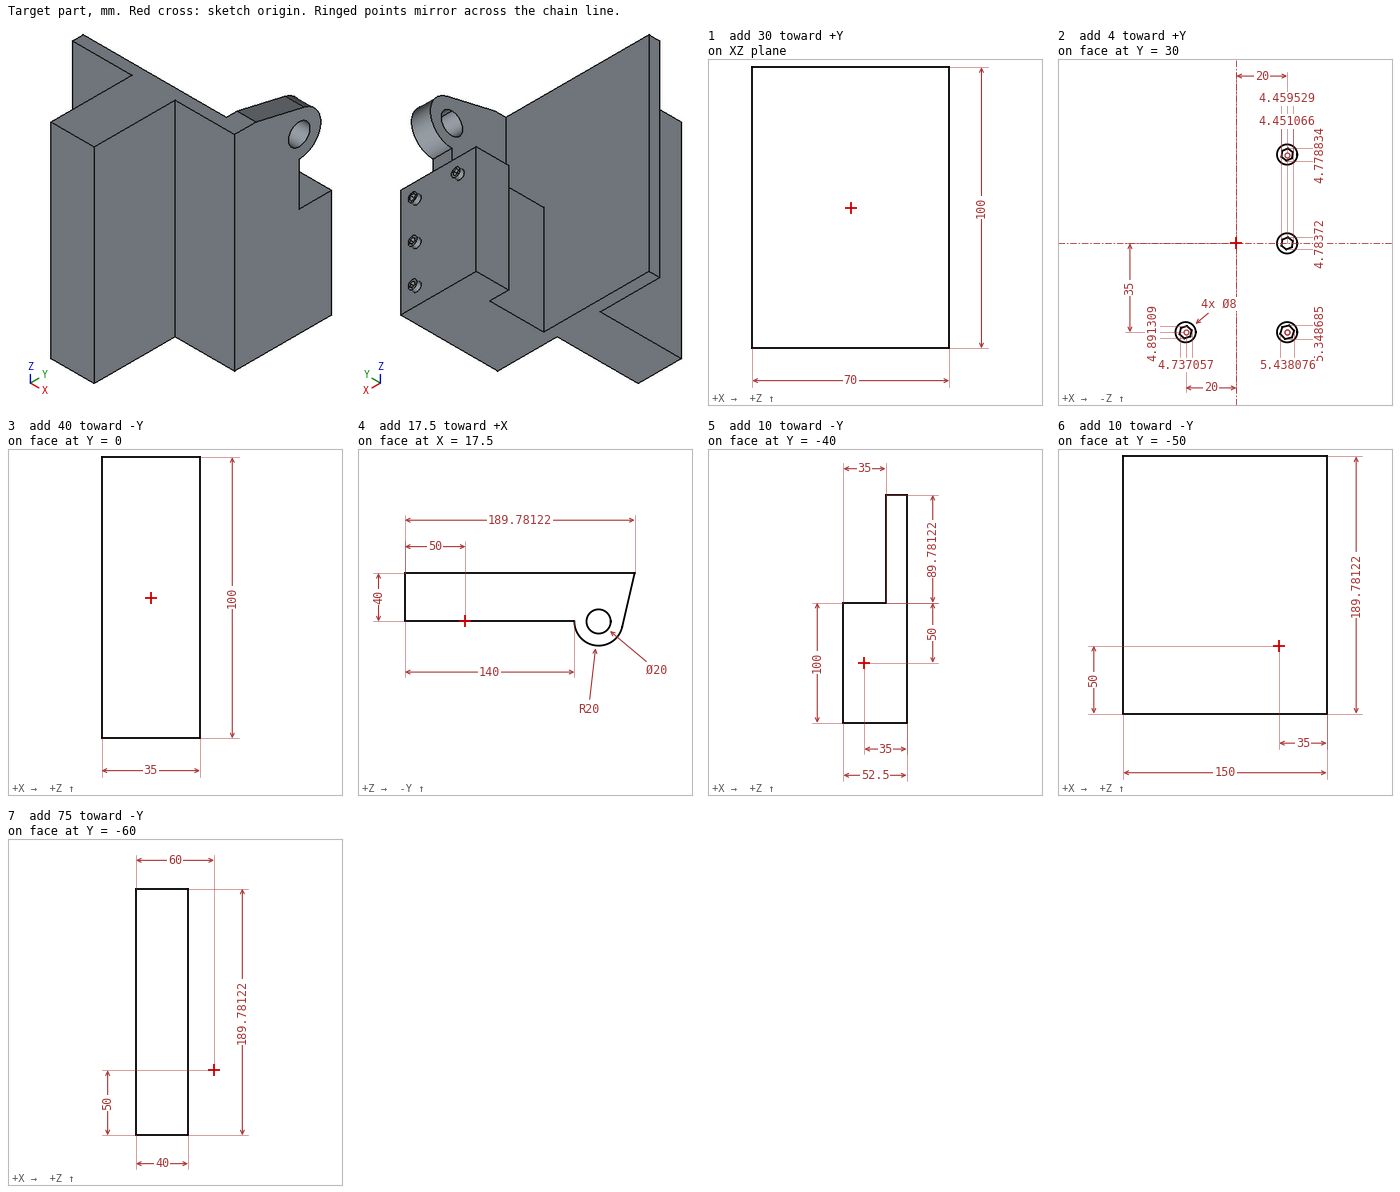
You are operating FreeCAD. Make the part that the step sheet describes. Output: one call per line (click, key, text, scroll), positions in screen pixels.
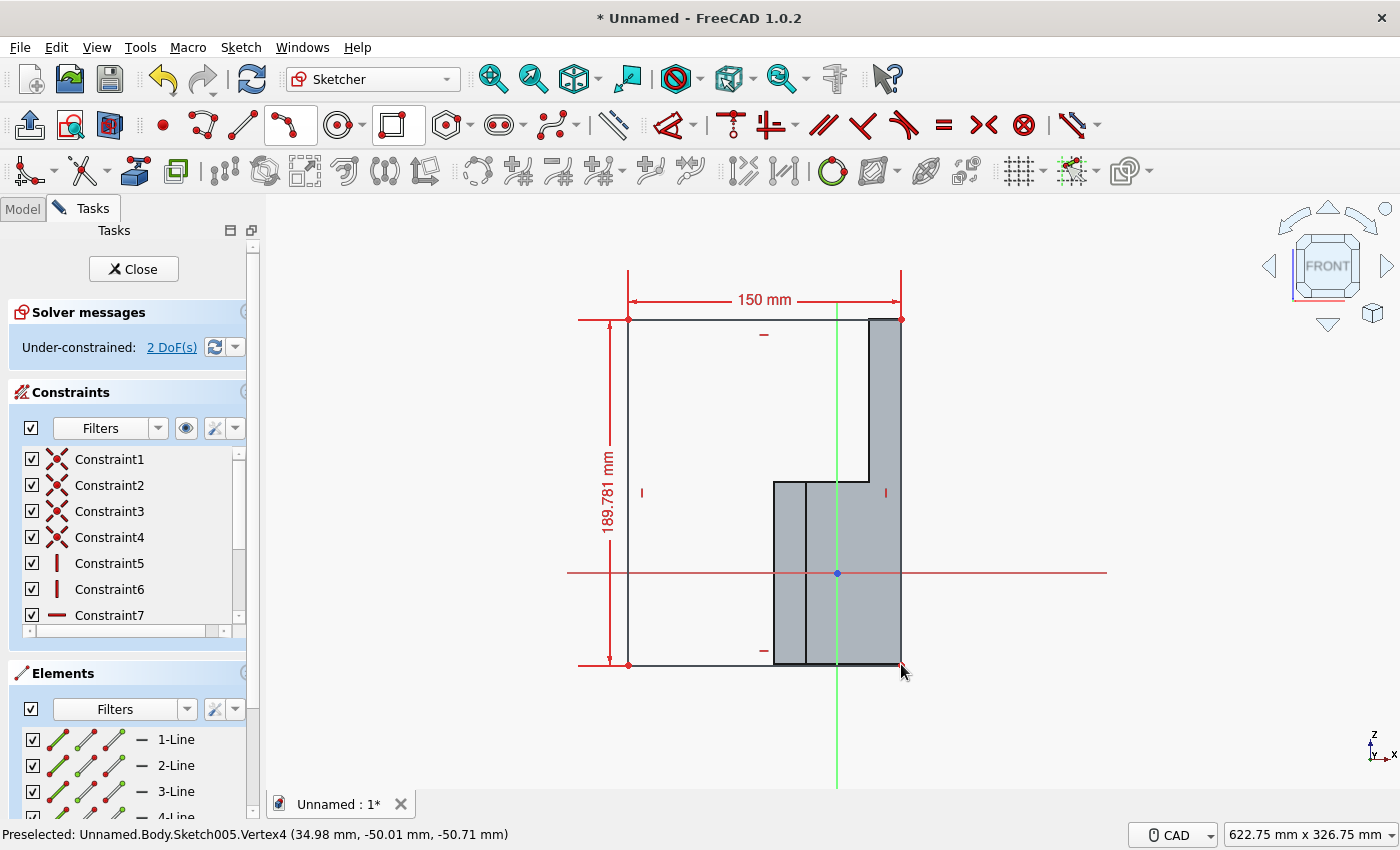
key(d)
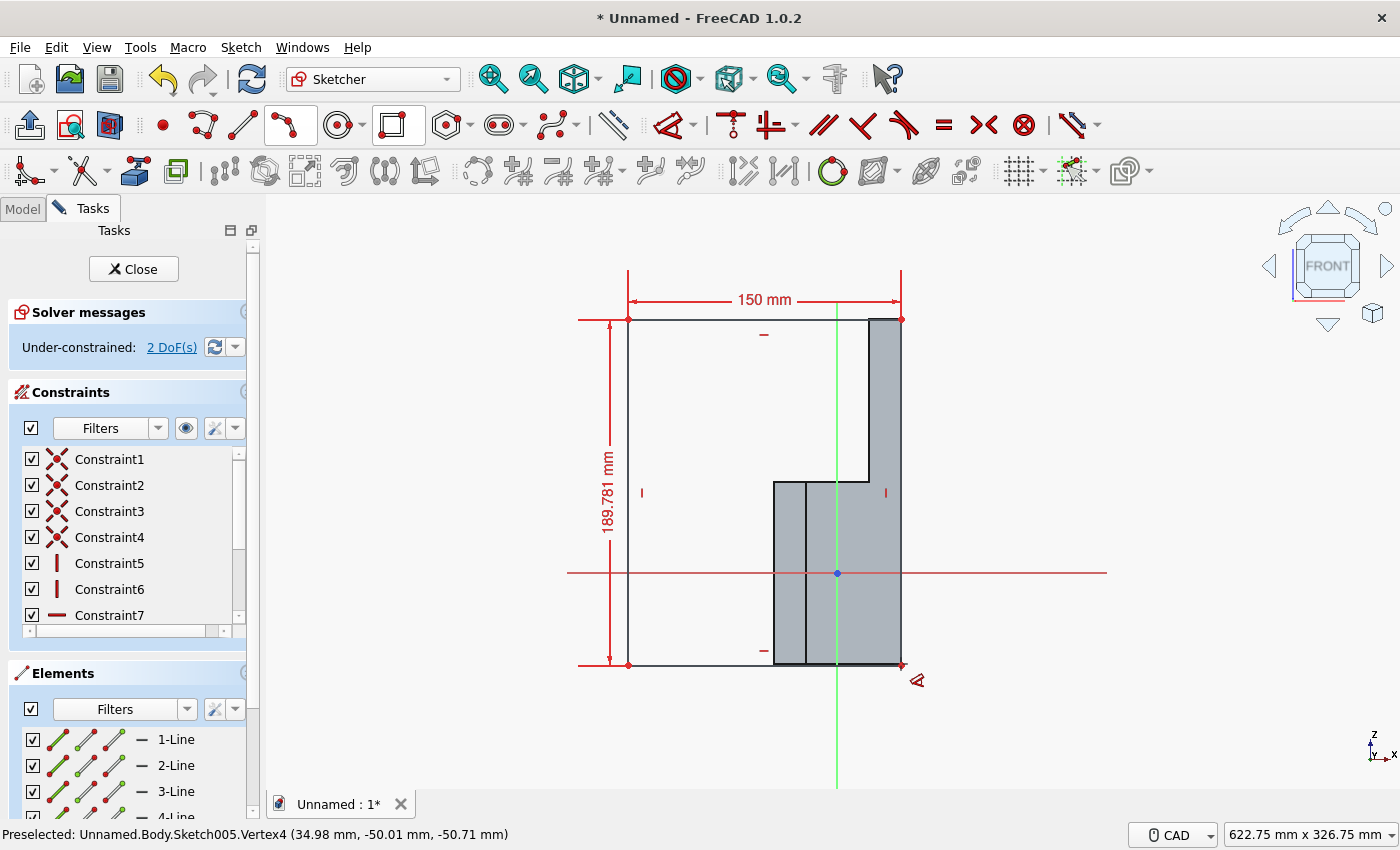
click(628, 666)
click(594, 619)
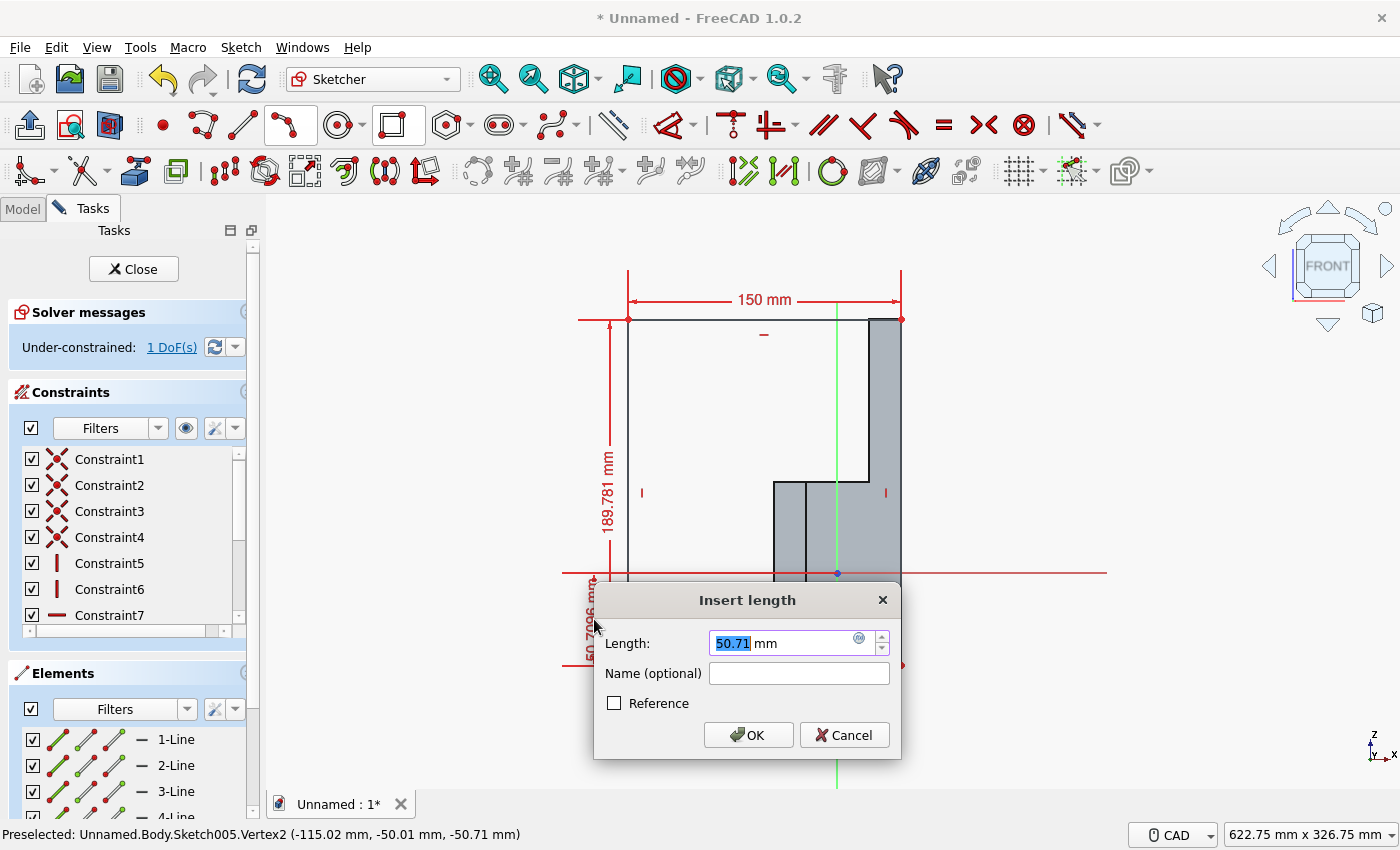
text(50)
key(Return)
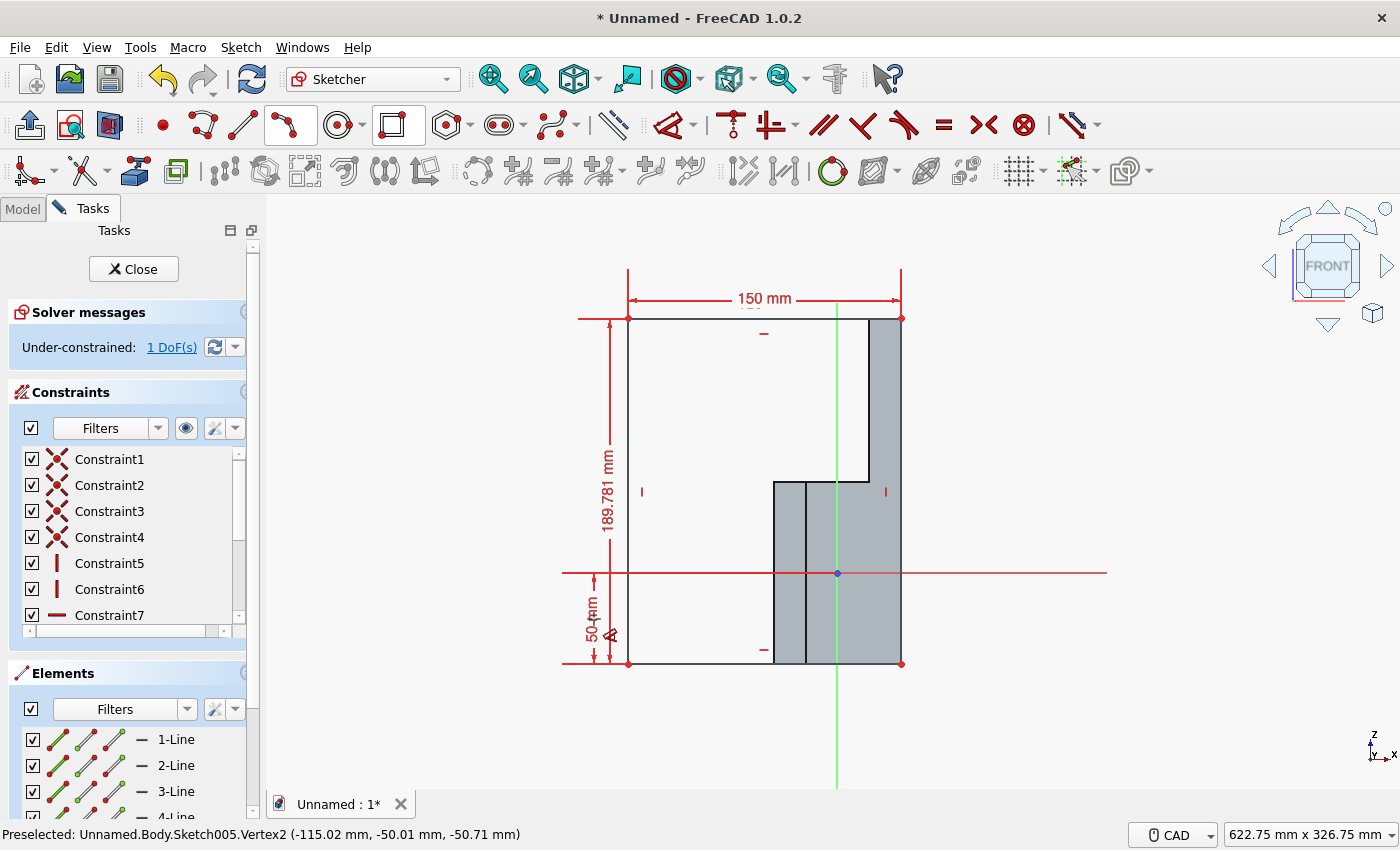
click(901, 664)
click(869, 698)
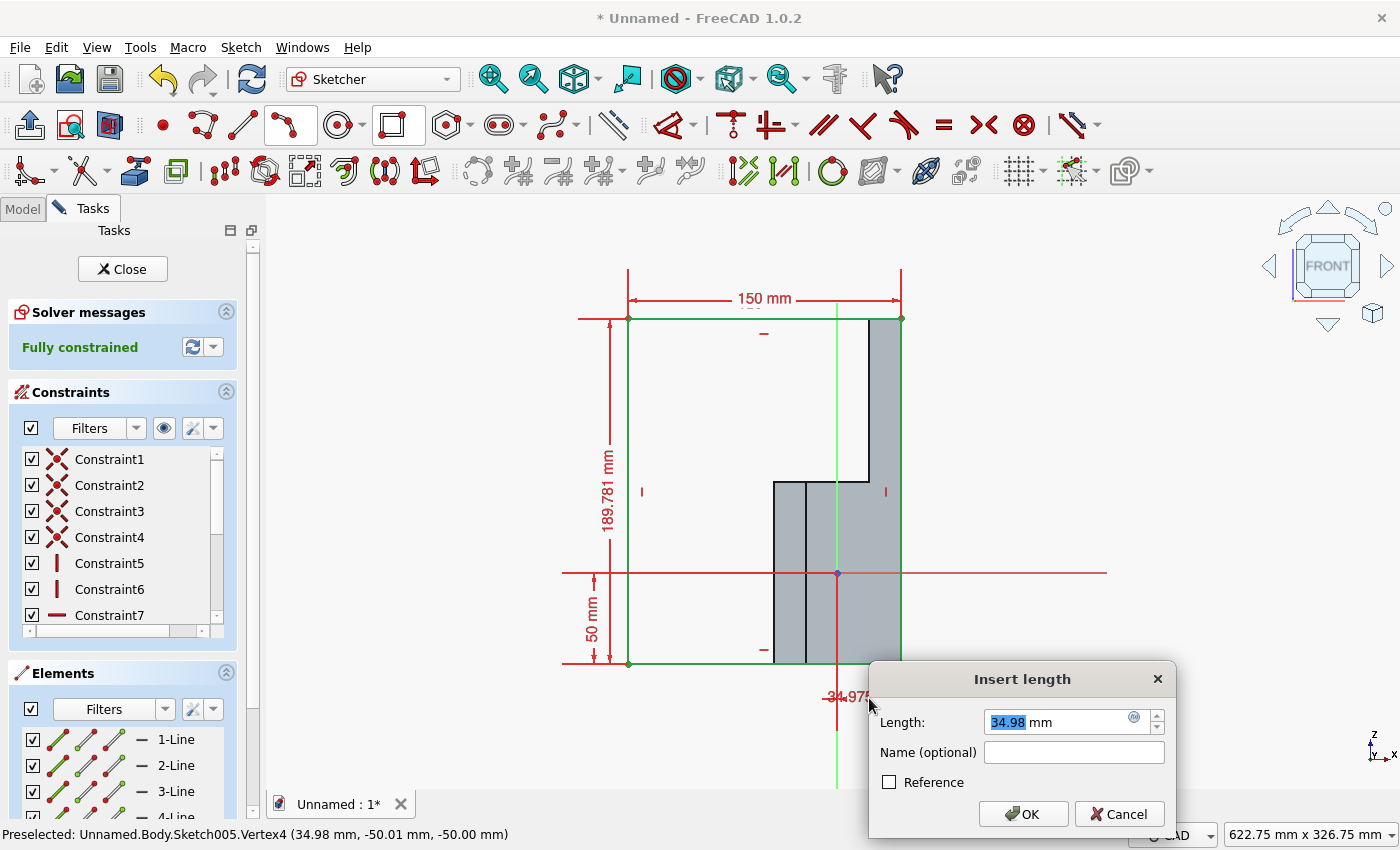
text(35)
key(Return)
key(Escape)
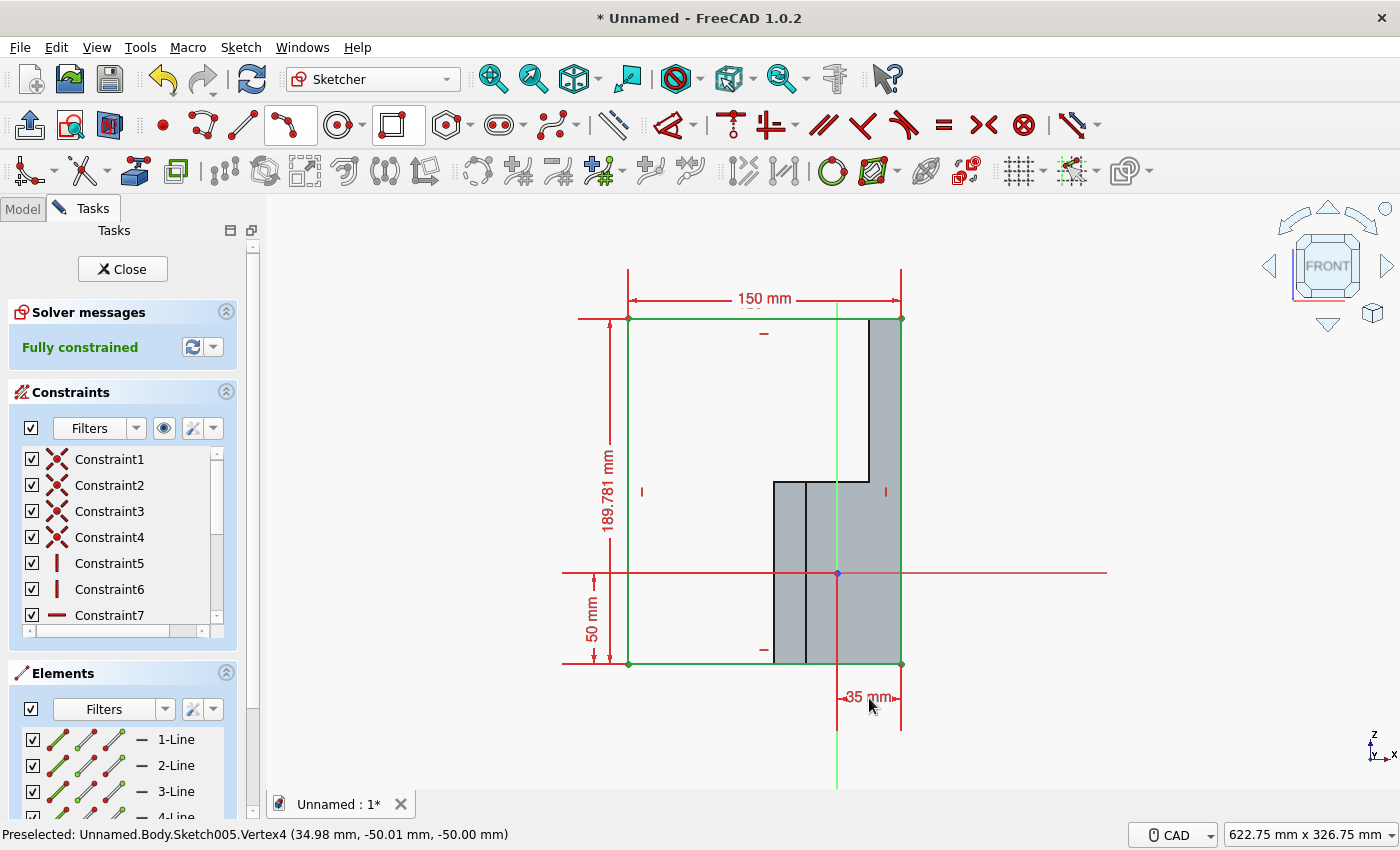
click(123, 269)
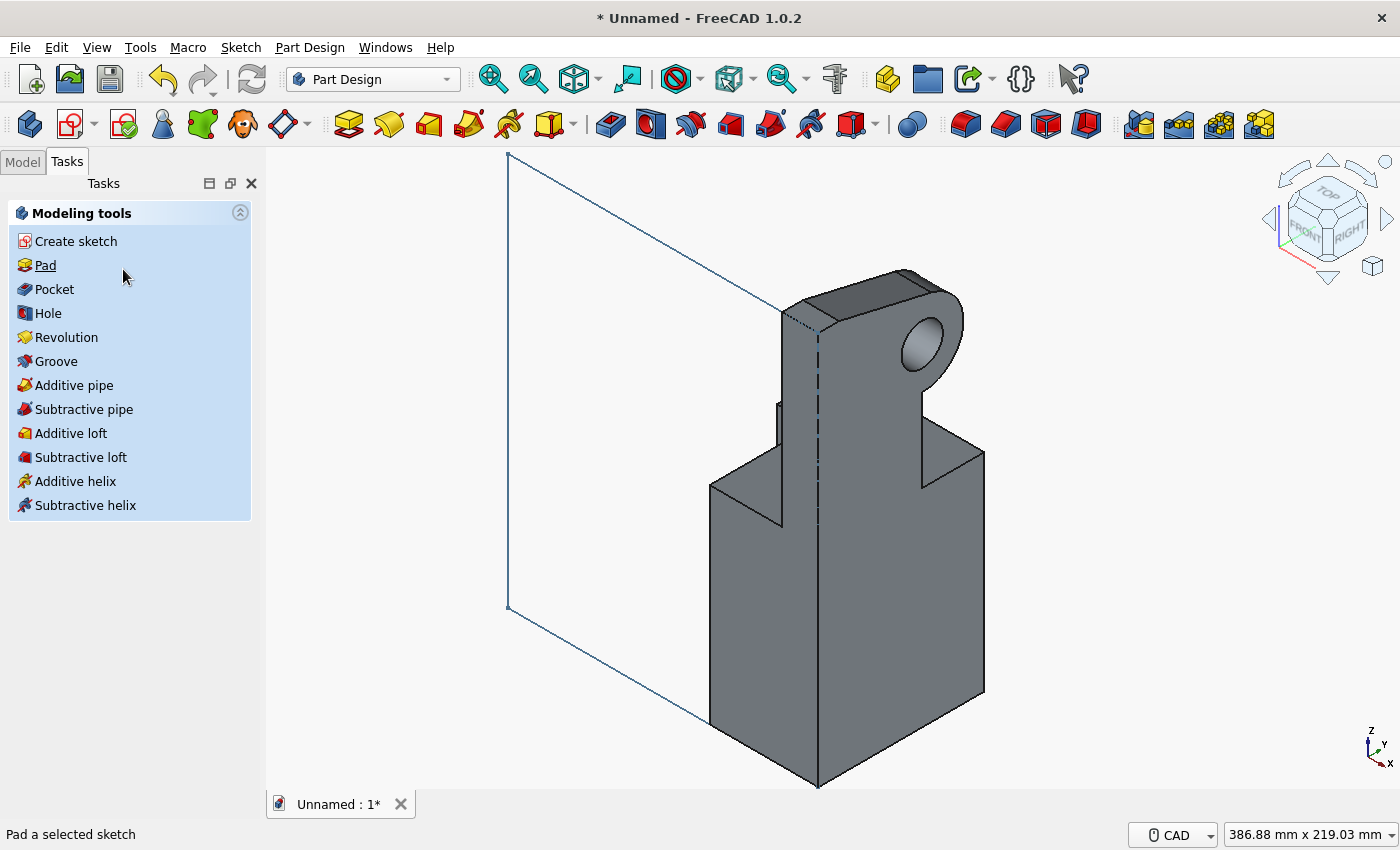
click(350, 124)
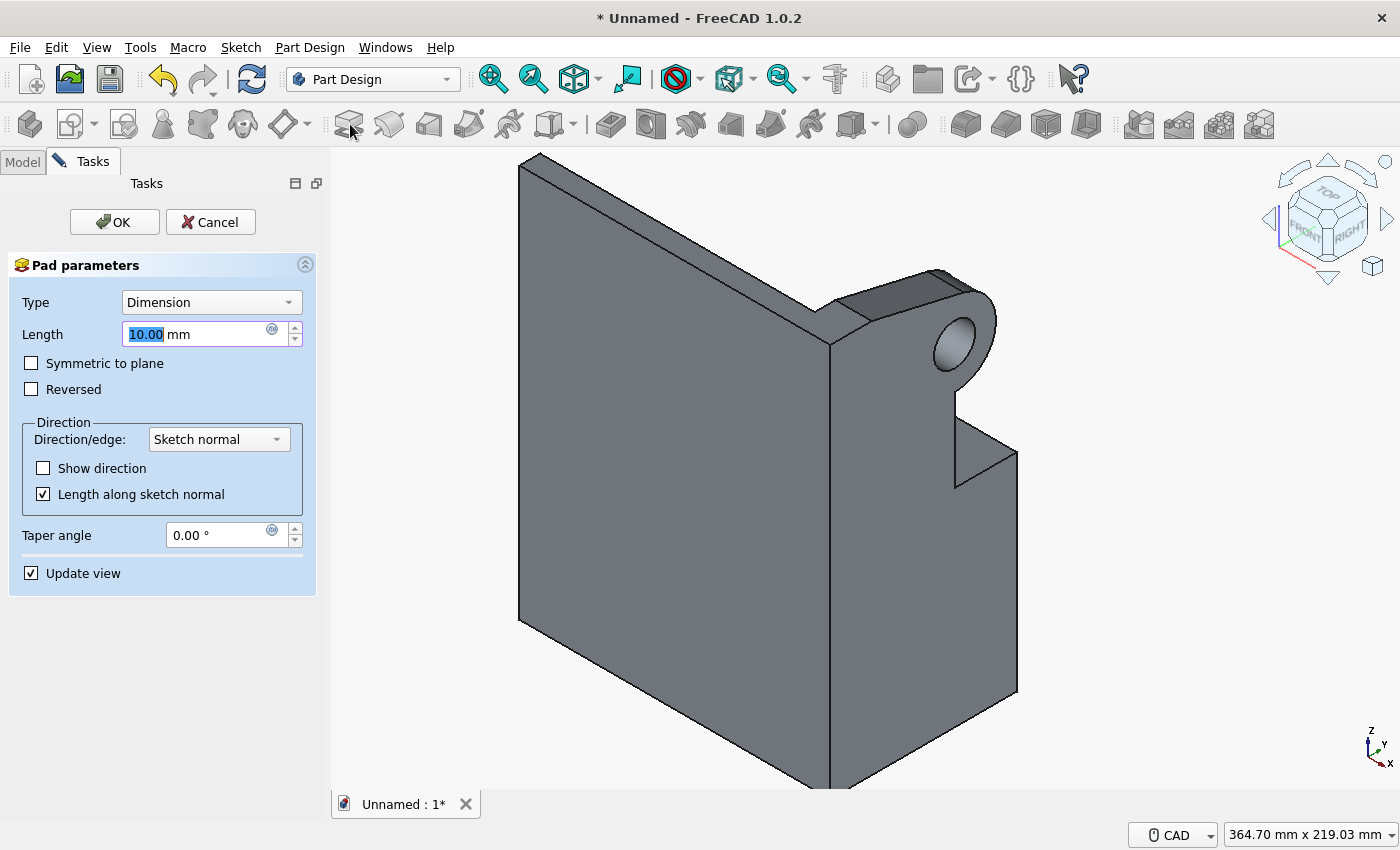
text(10)
key(Tab)